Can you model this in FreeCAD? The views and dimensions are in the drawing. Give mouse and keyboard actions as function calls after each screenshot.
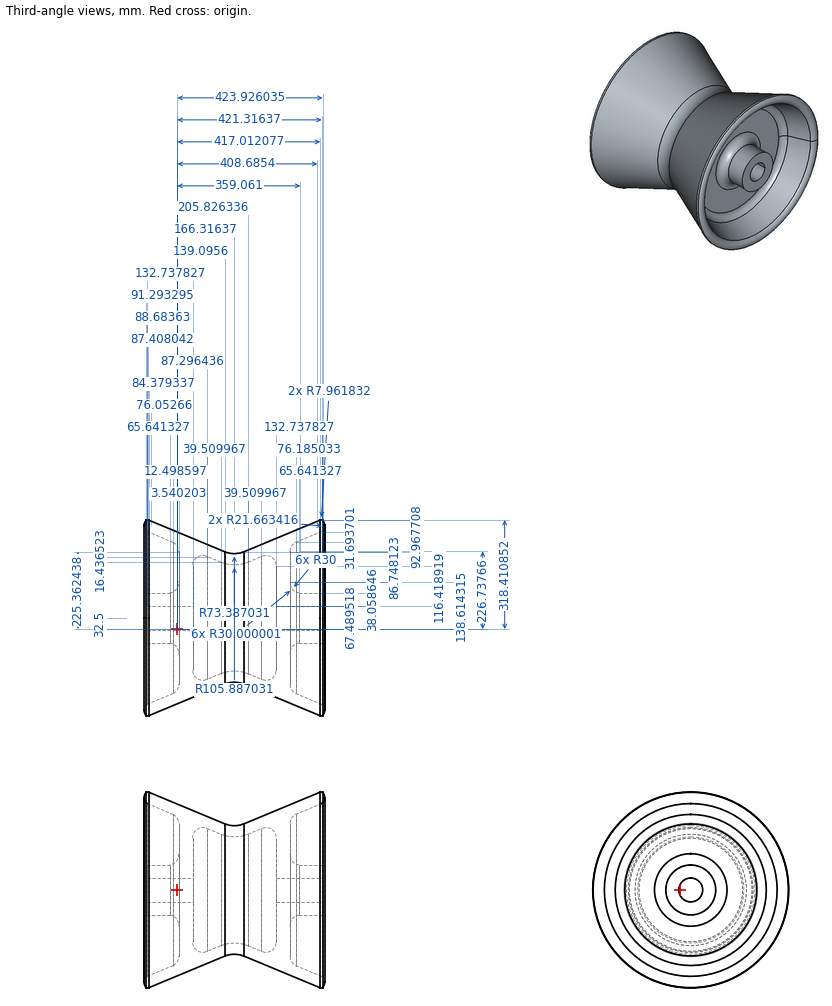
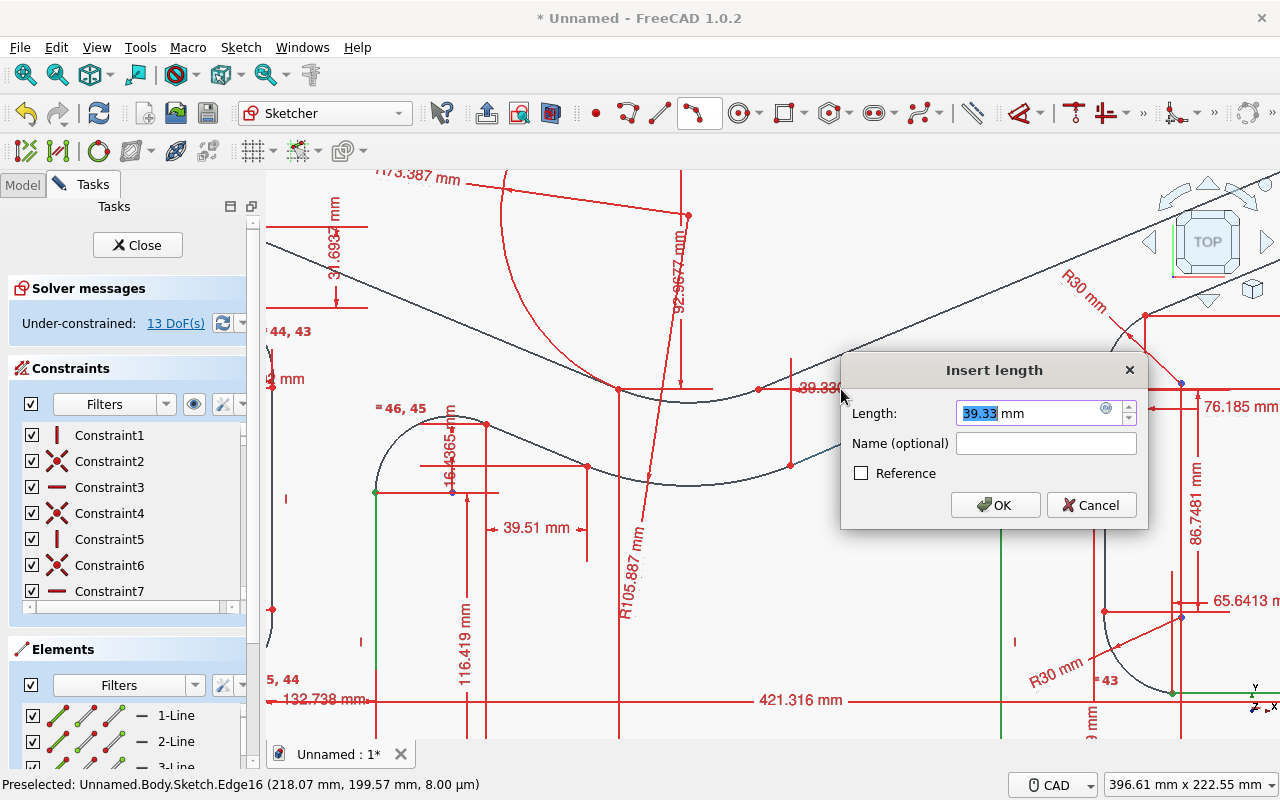
text(39.509967)
key(Return)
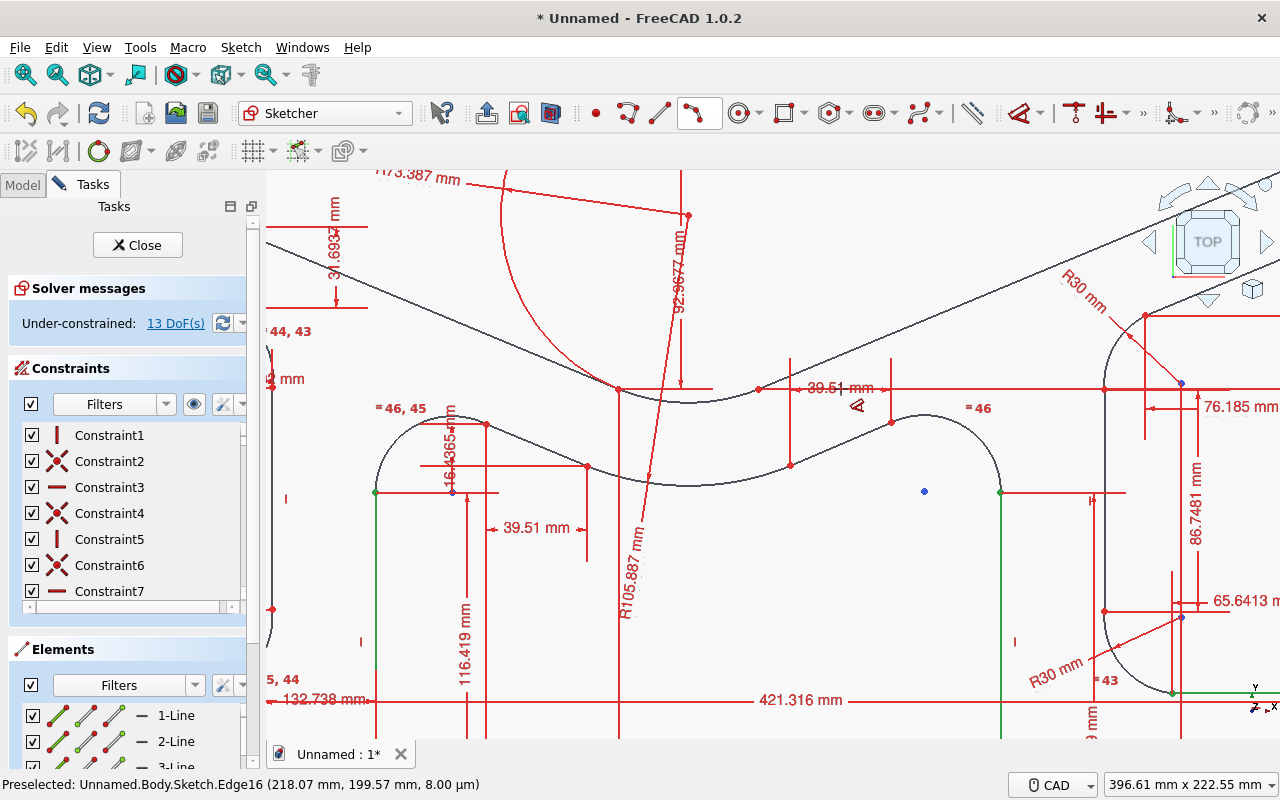
click(821, 453)
click(925, 444)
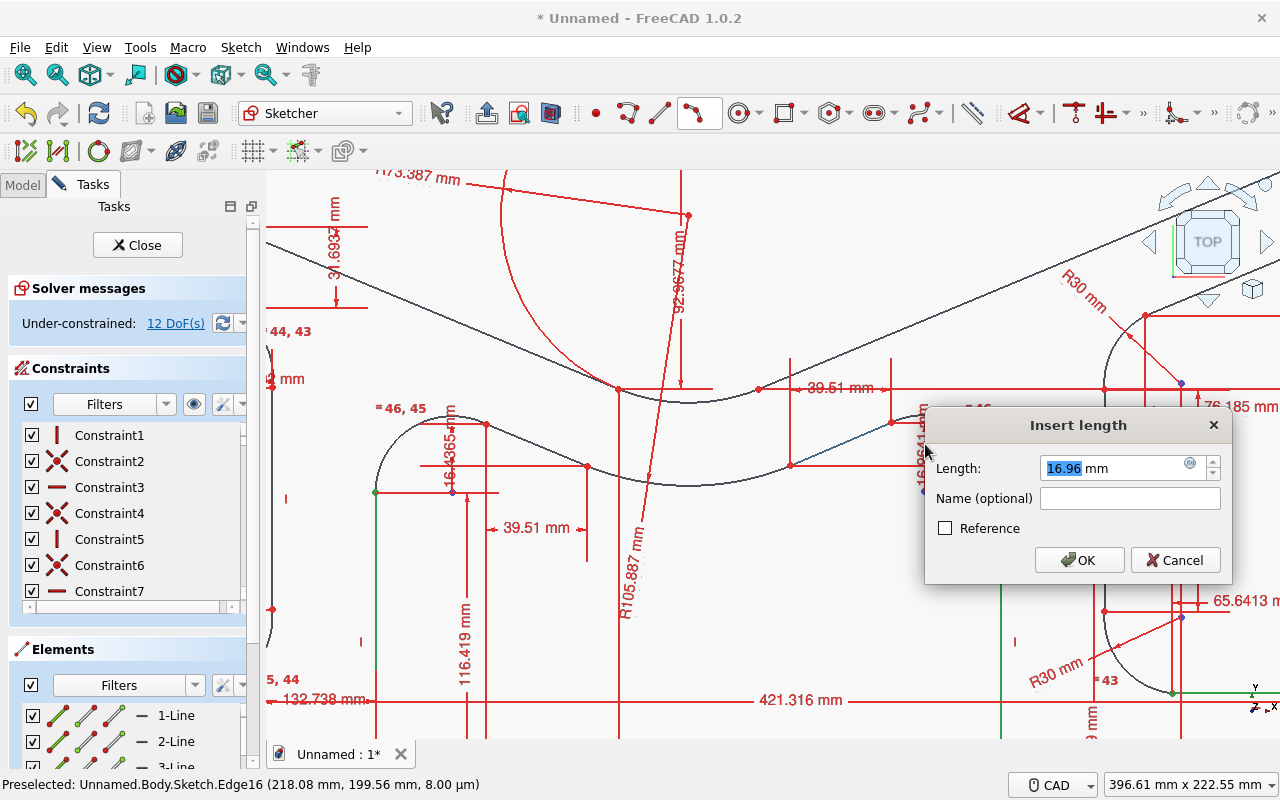
text(16.436523)
key(Return)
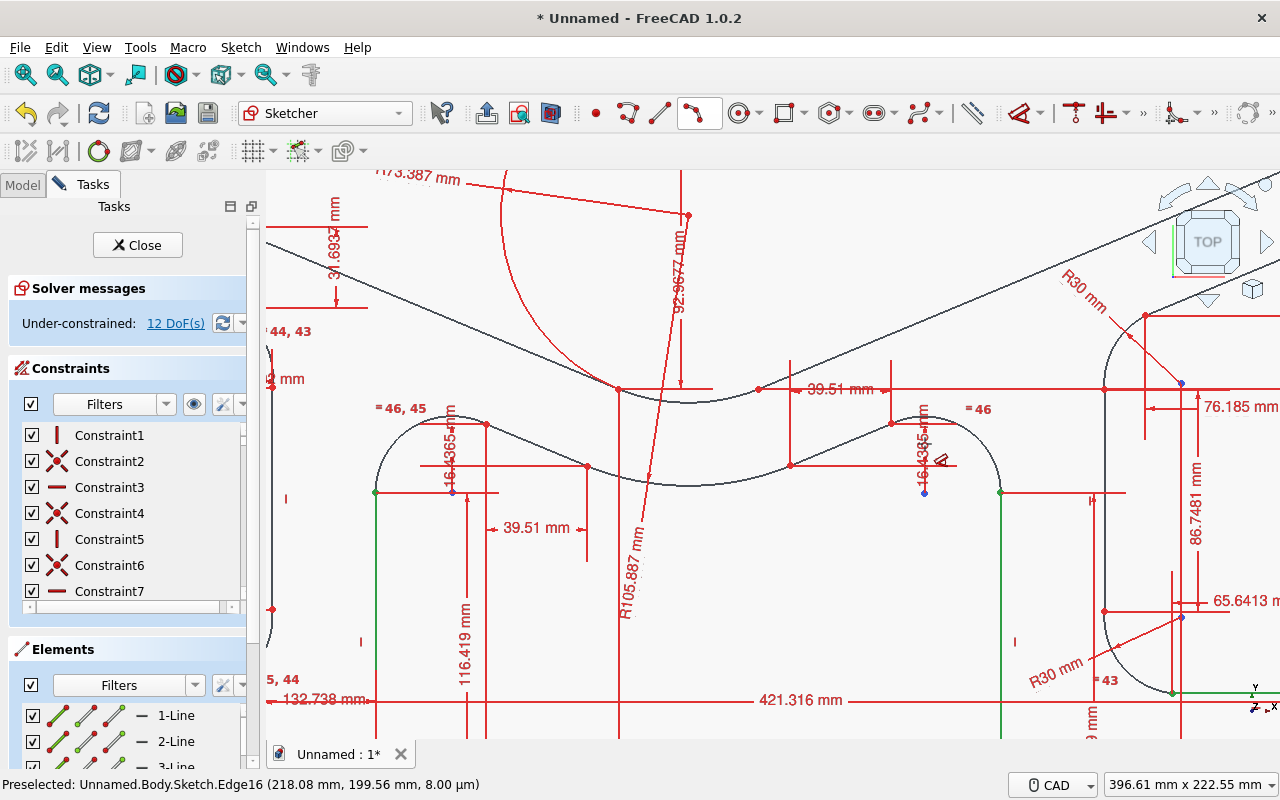
scroll(714, 396, down, 5)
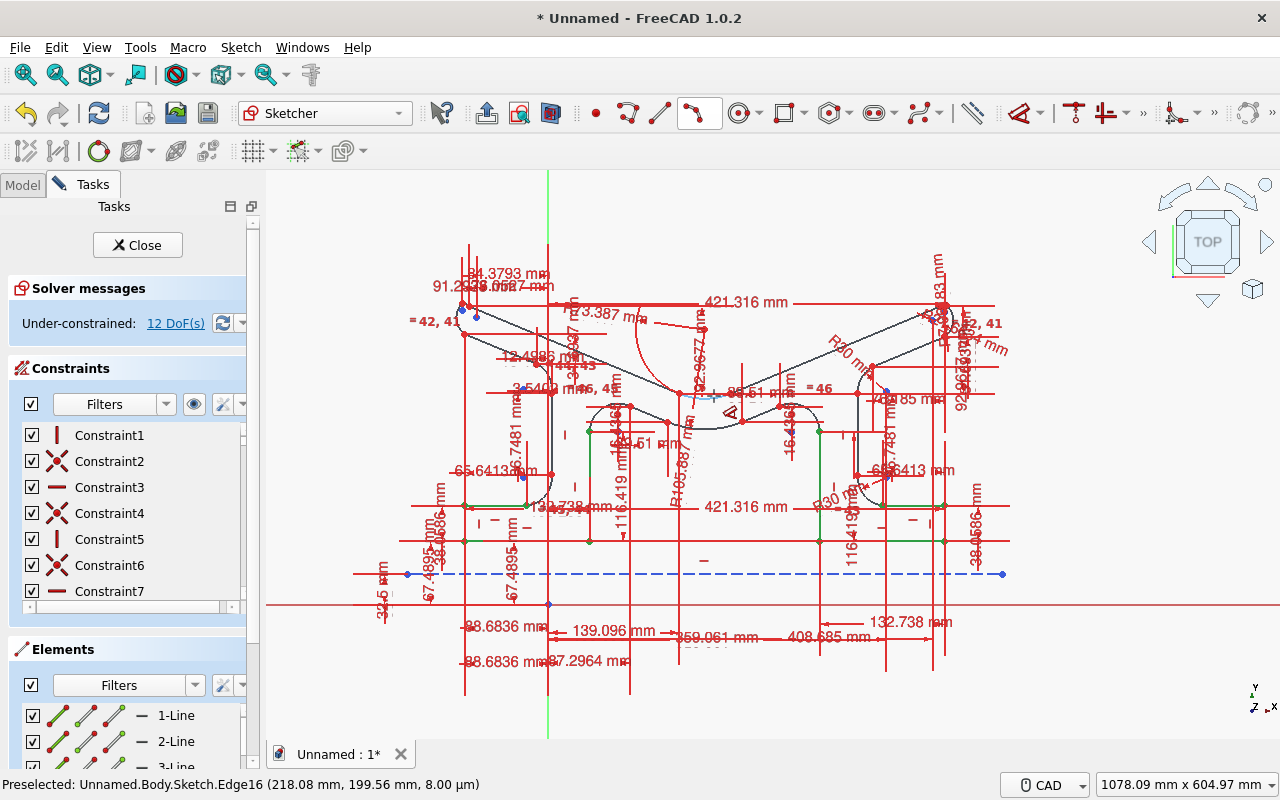
click(886, 392)
click(968, 498)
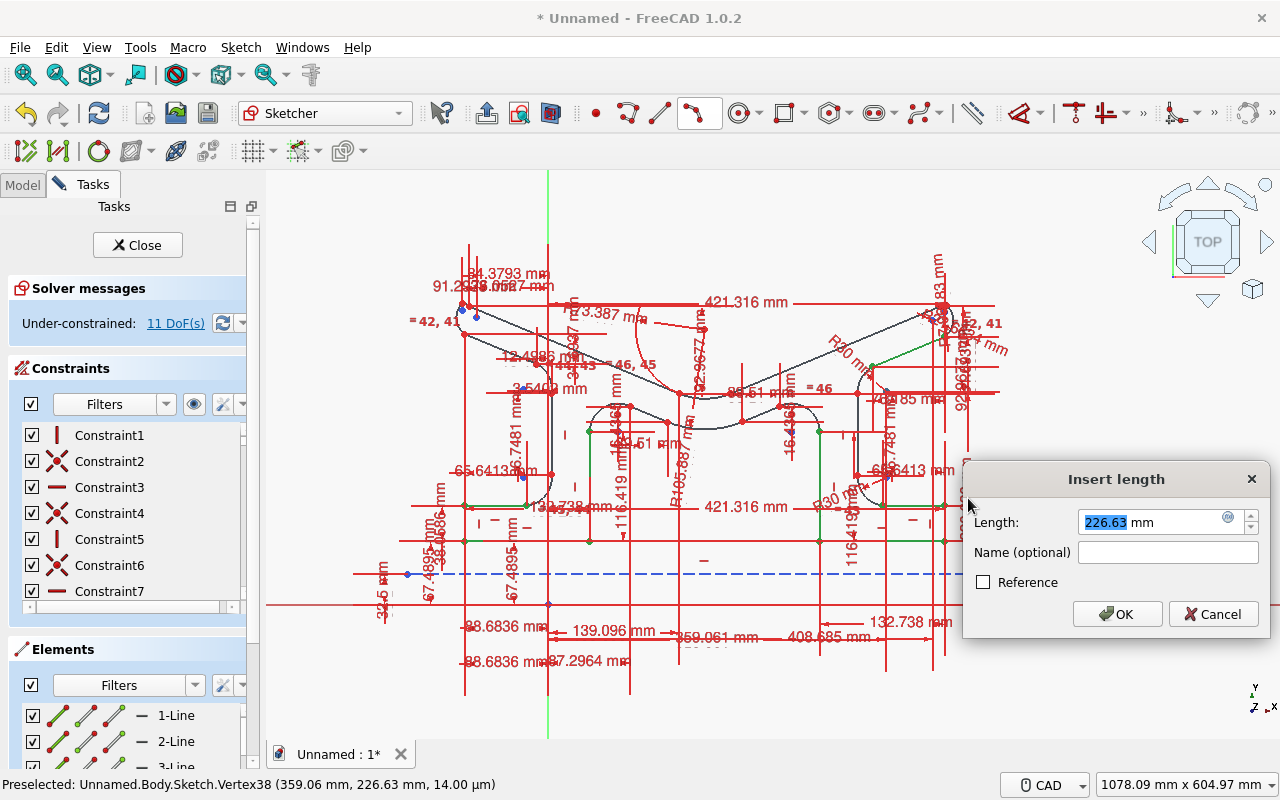
text(226.73766)
key(Return)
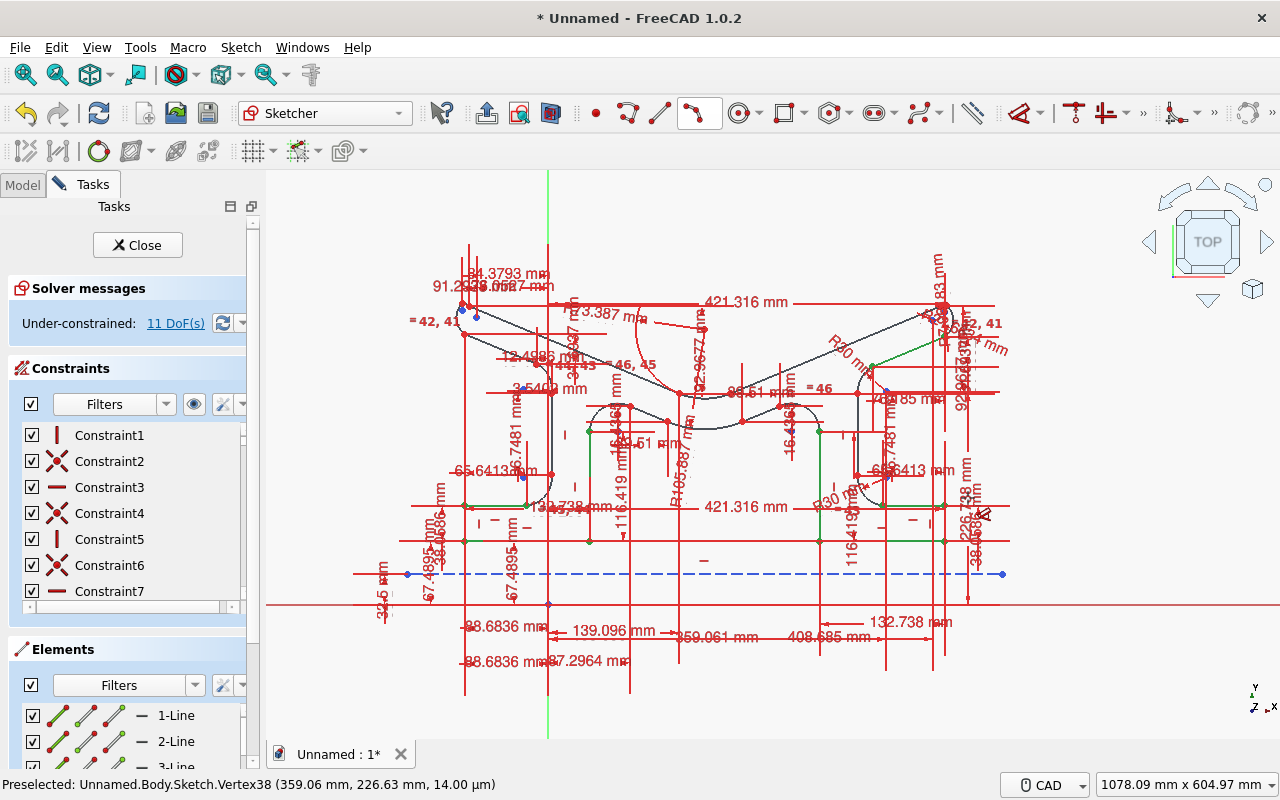
click(705, 330)
click(663, 663)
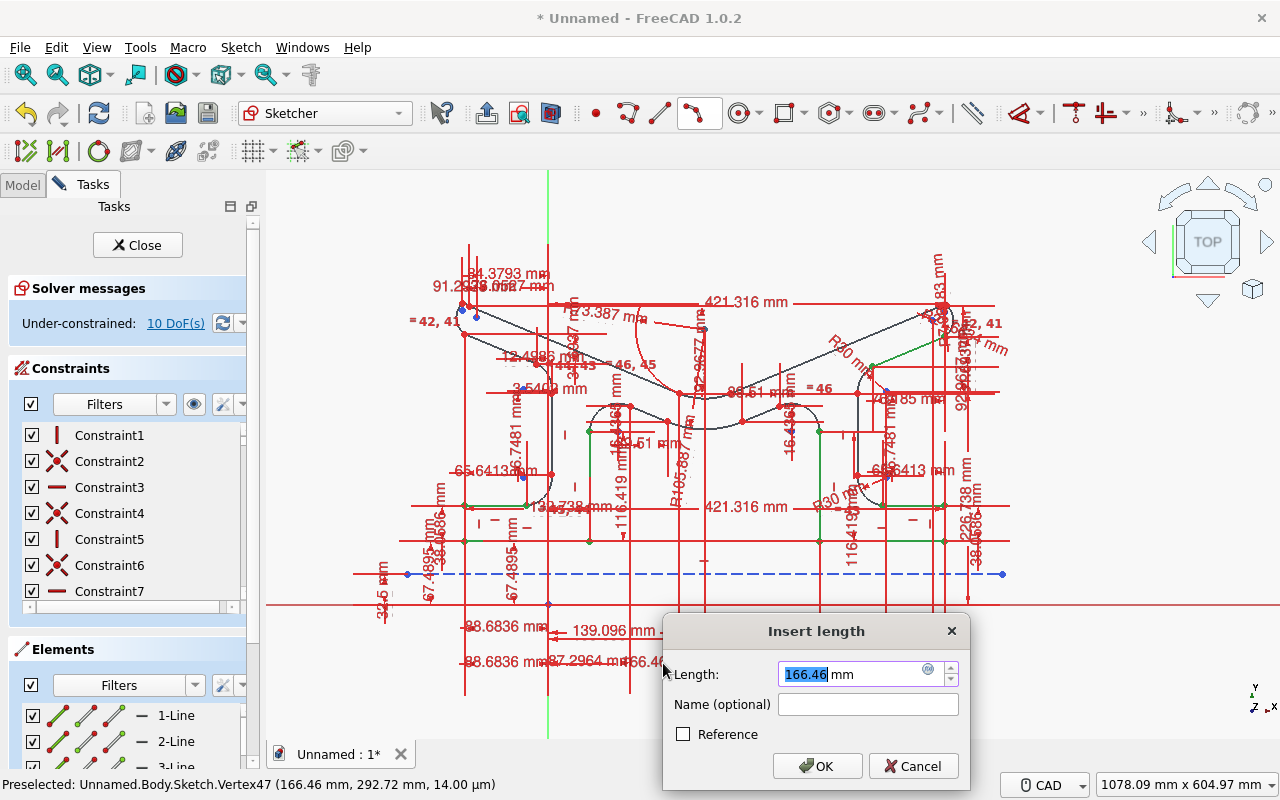
text(166.31637)
key(Return)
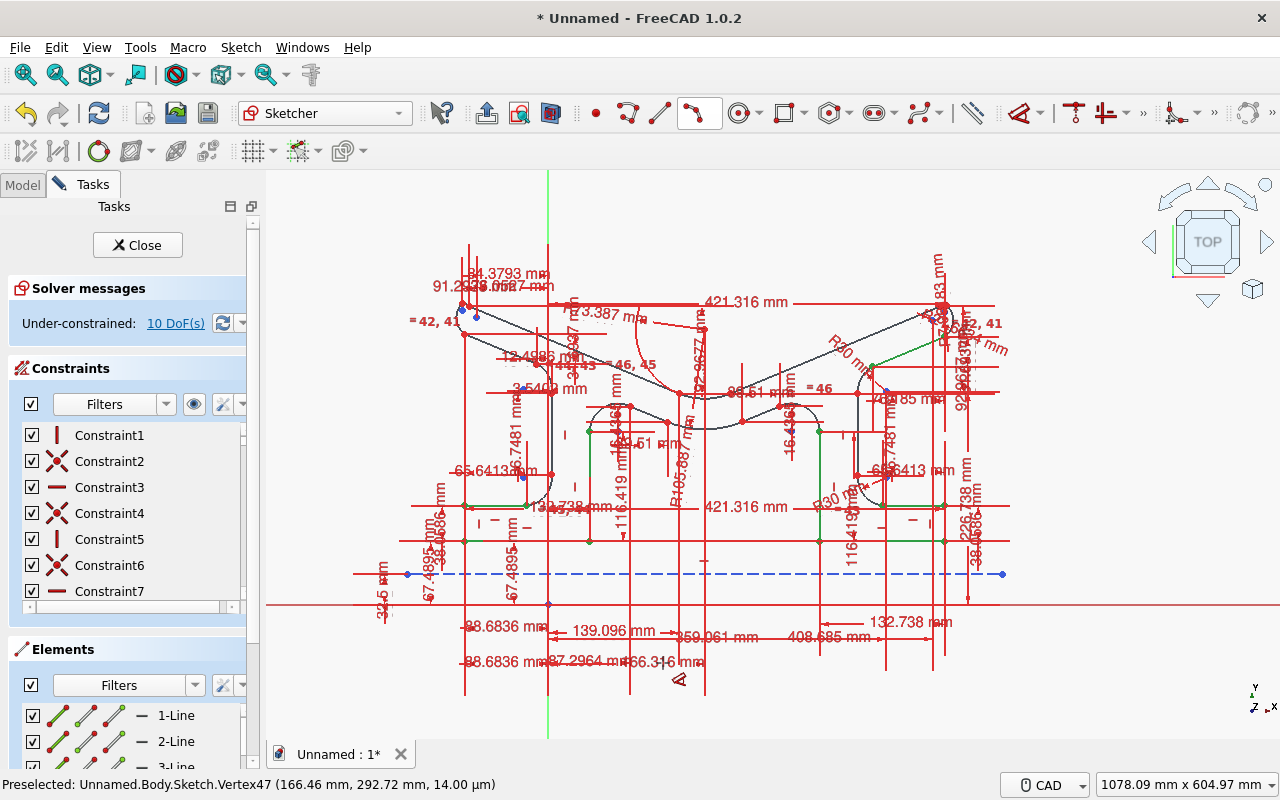
scroll(463, 311, up, 3)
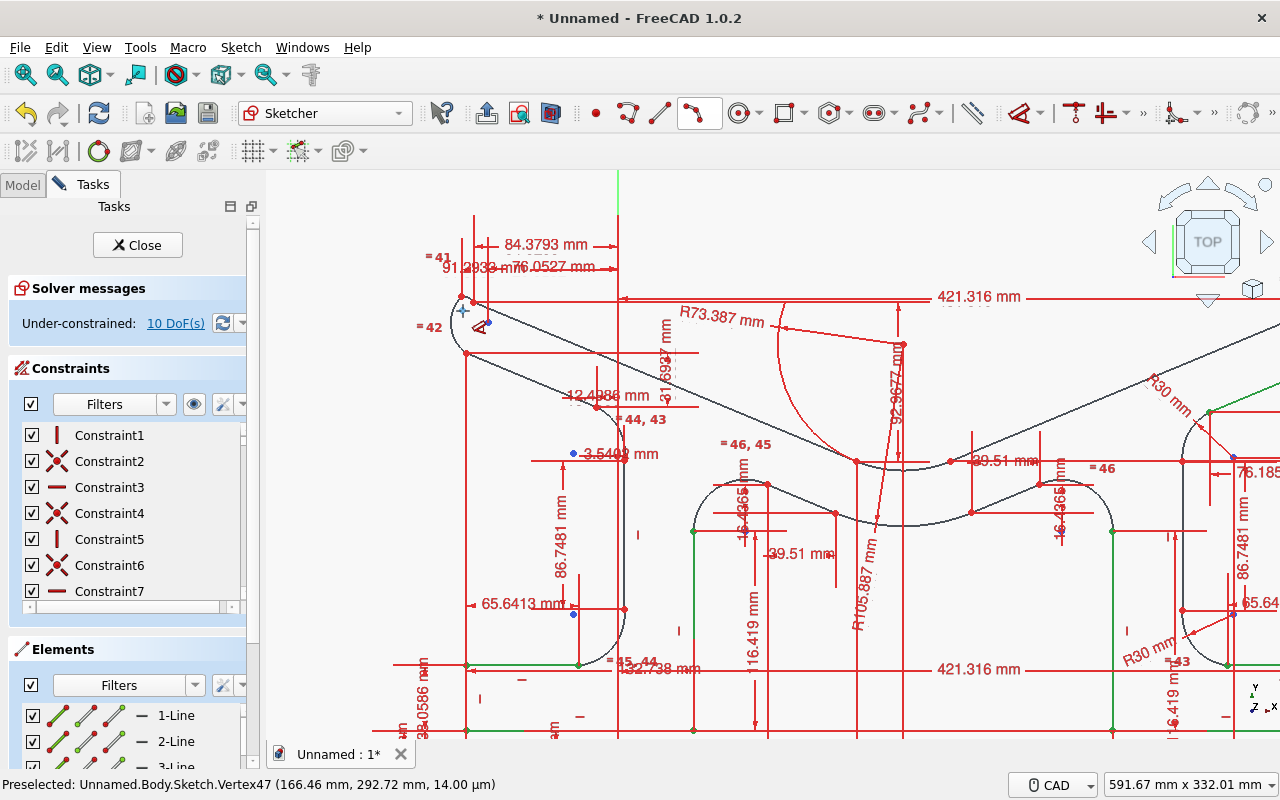
click(463, 310)
click(541, 204)